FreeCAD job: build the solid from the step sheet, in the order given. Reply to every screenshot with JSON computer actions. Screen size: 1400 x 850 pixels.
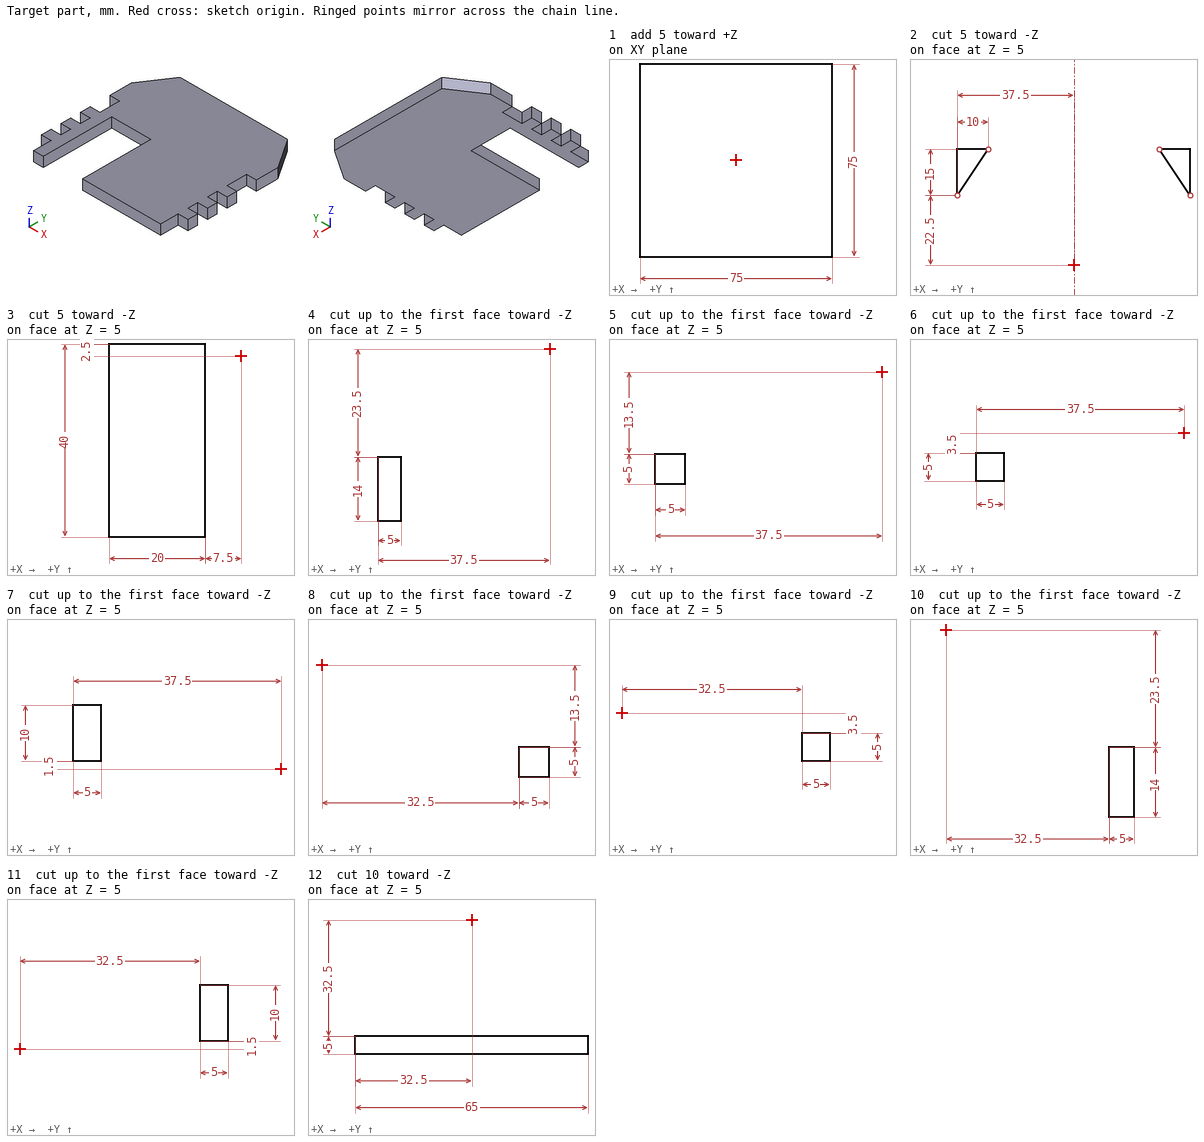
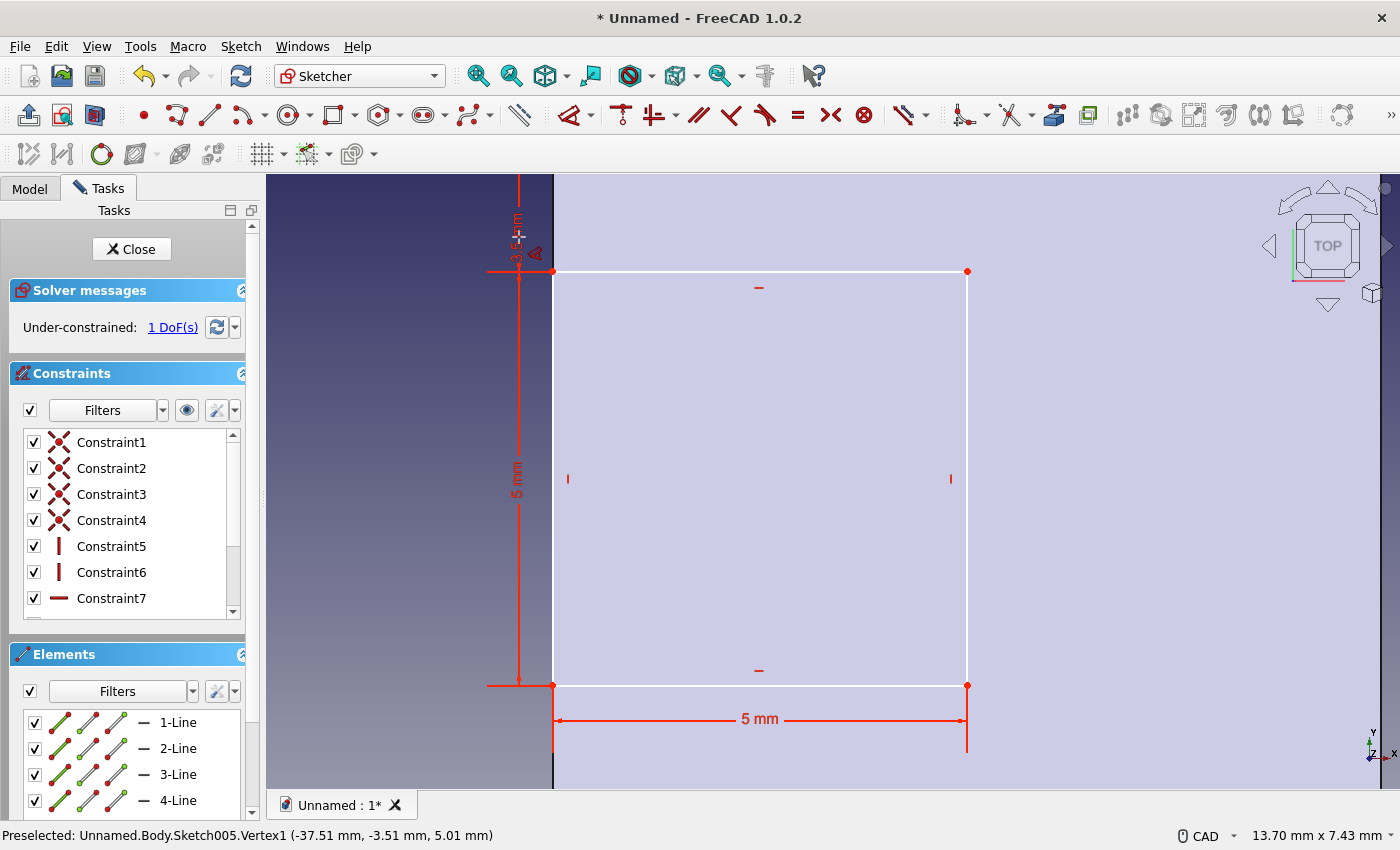
{"action": "left_click", "coordinate": [553, 272]}
{"action": "left_click", "coordinate": [894, 306]}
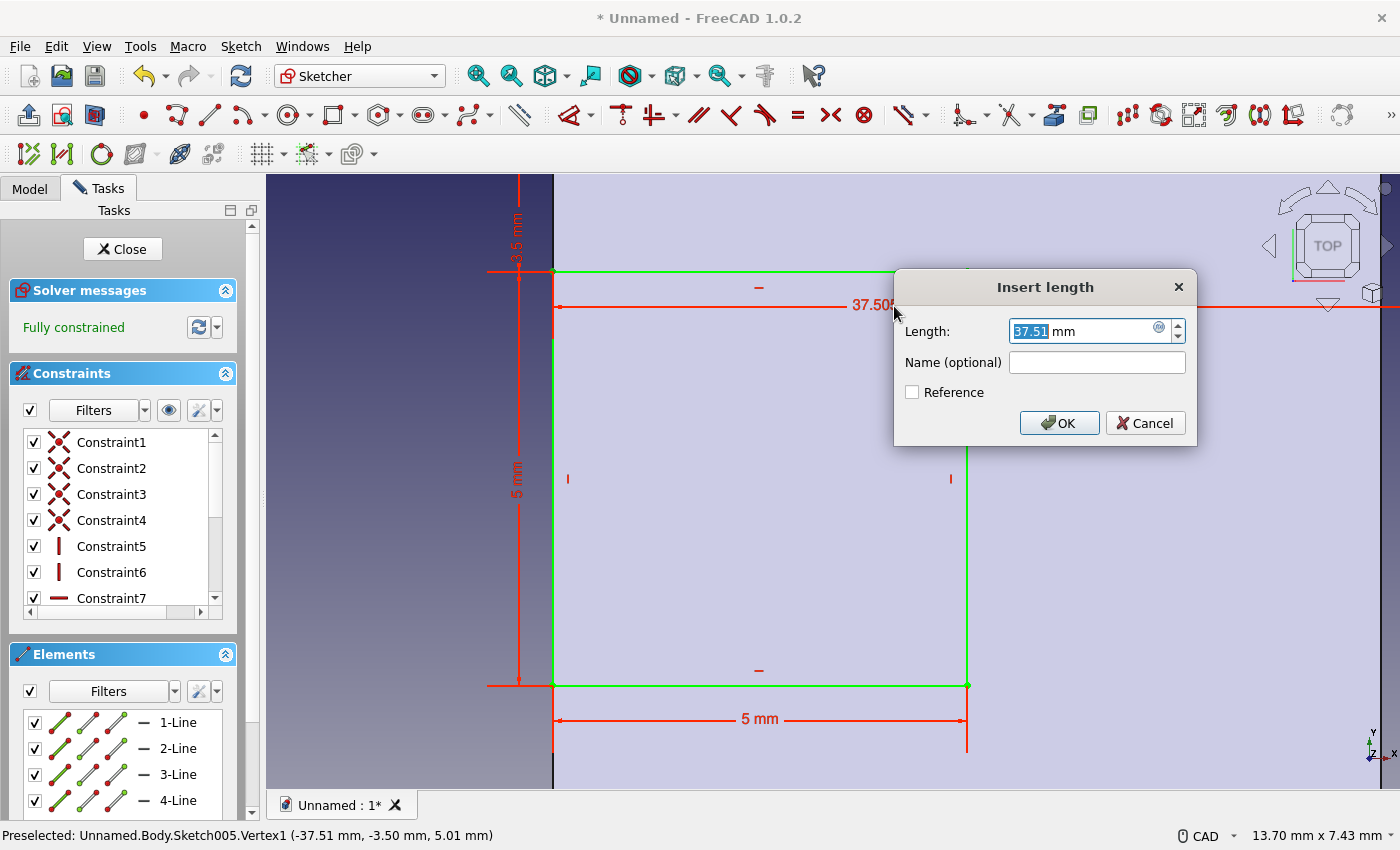
{"action": "type", "text": "37.5"}
{"action": "key", "text": "Return"}
{"action": "key", "text": "Escape"}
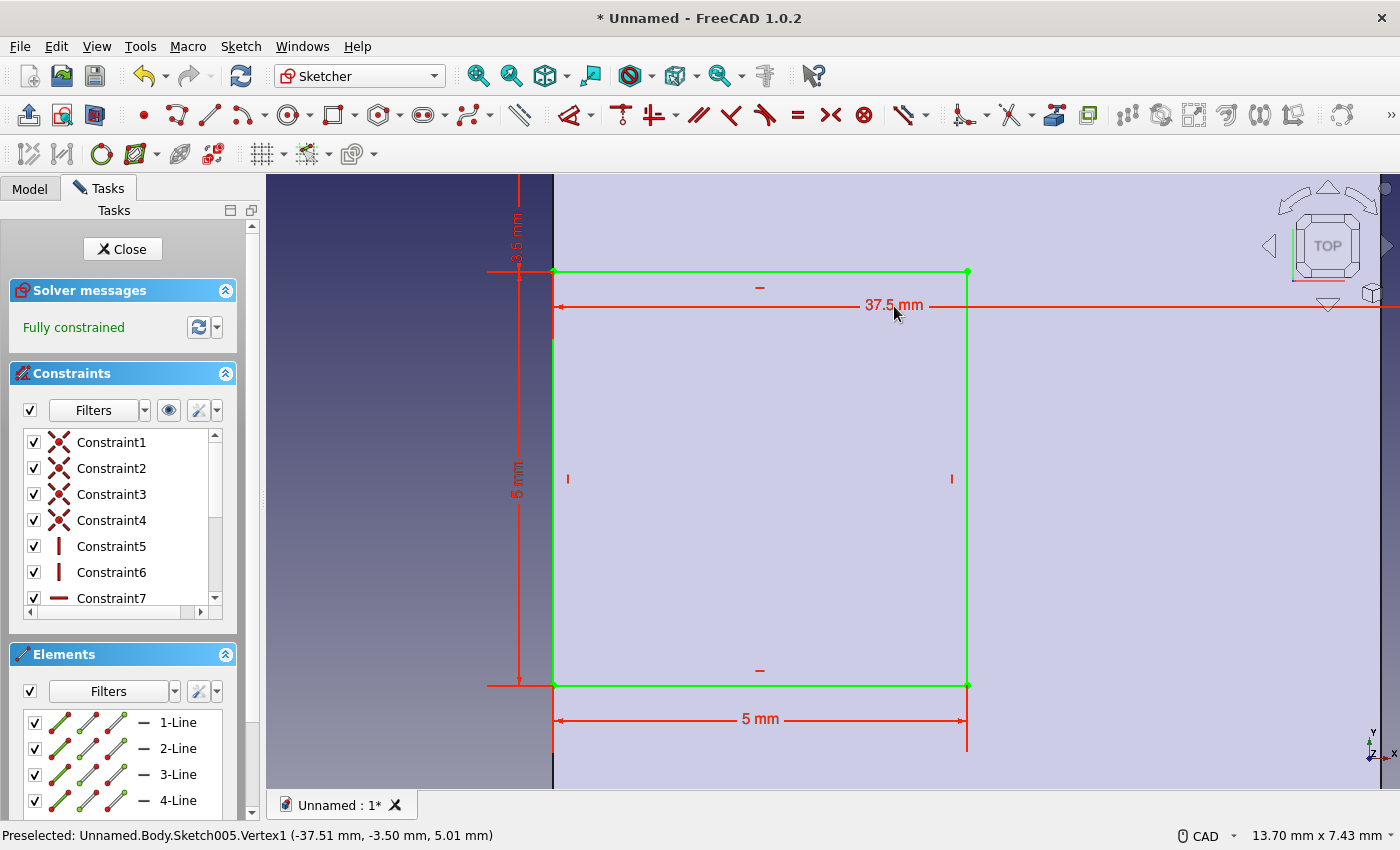
{"action": "left_click", "coordinate": [123, 249]}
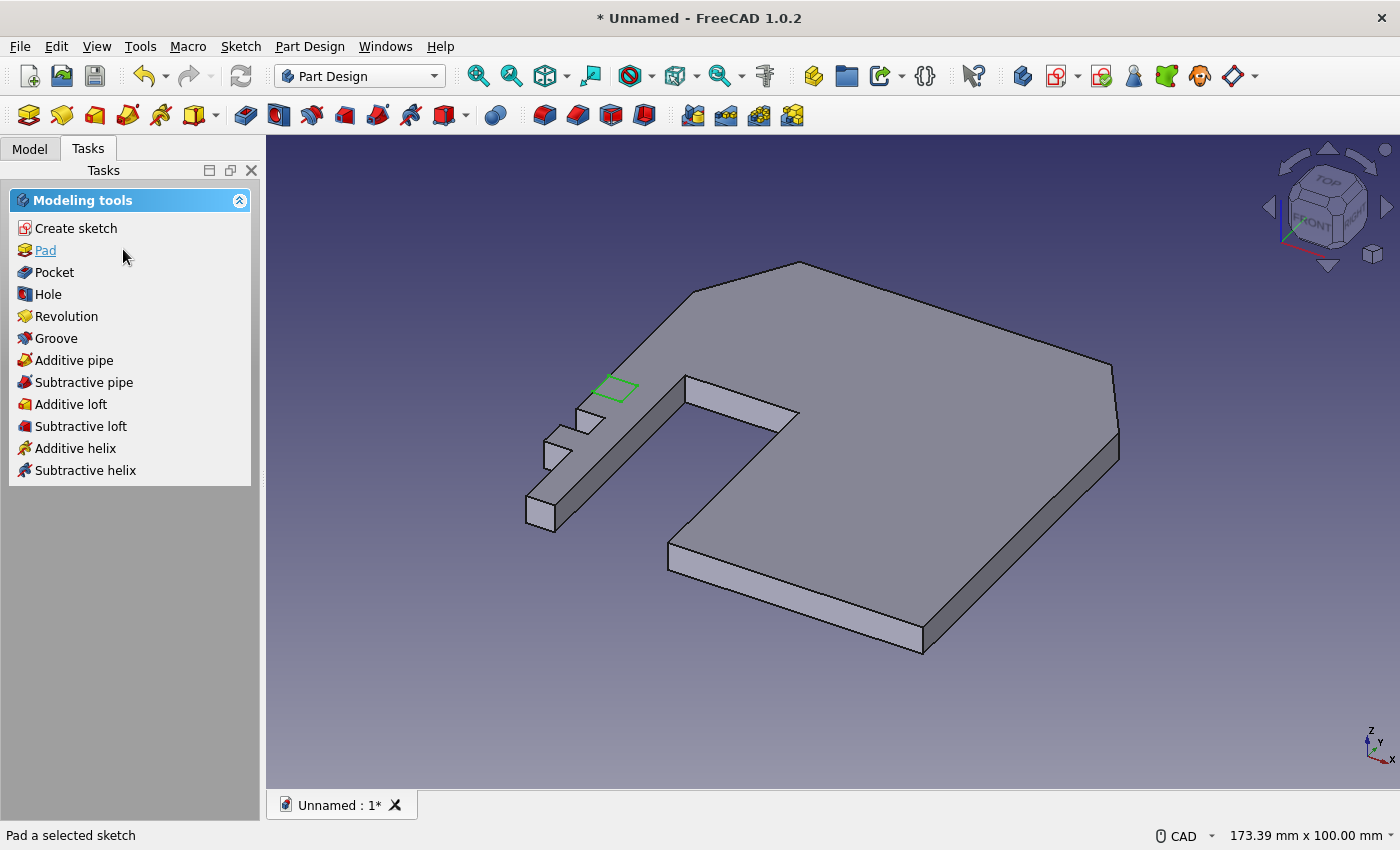
{"action": "left_click", "coordinate": [246, 116]}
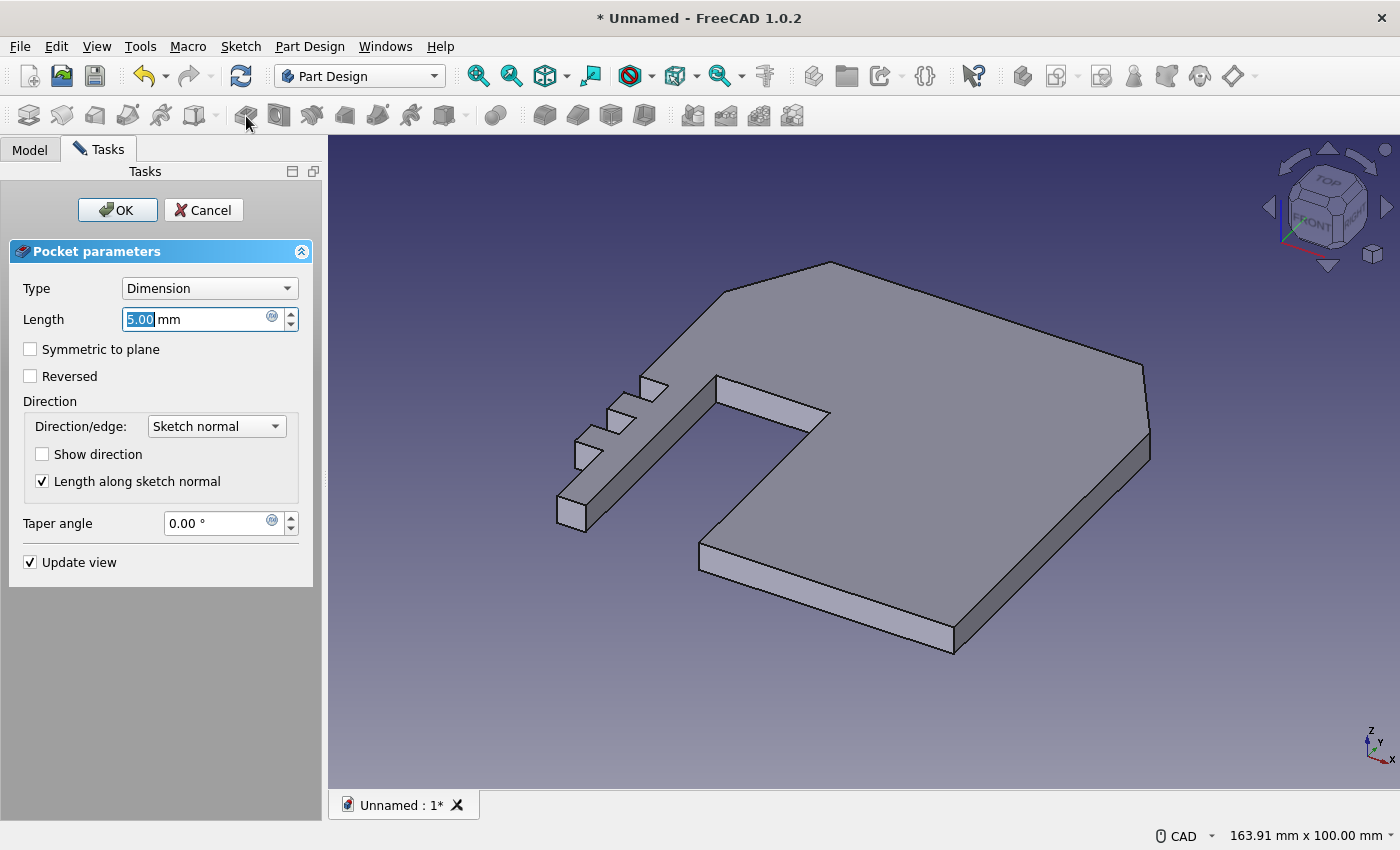
{"action": "left_click", "coordinate": [210, 288]}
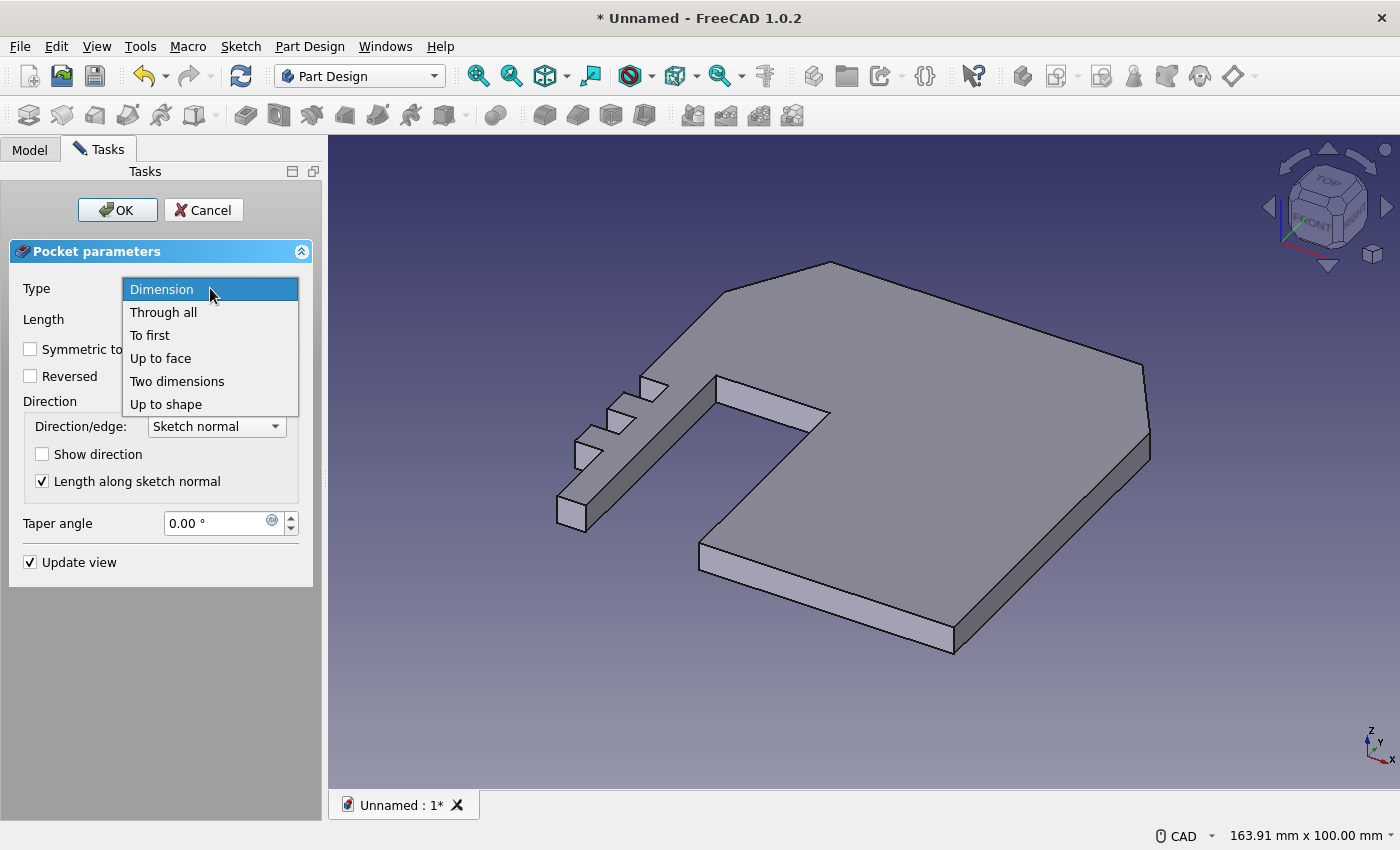
{"action": "left_click", "coordinate": [208, 336]}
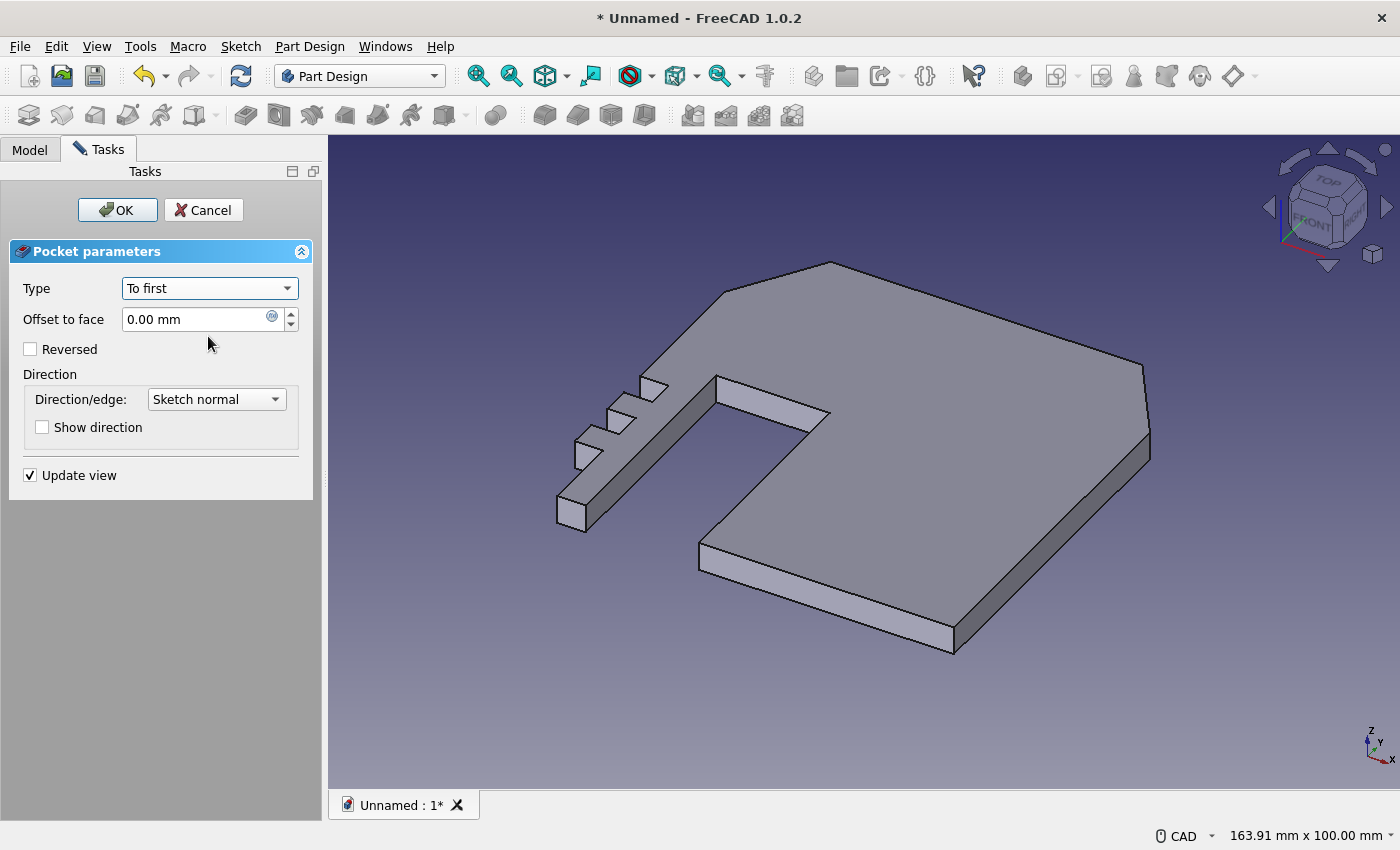
{"action": "left_click", "coordinate": [118, 210]}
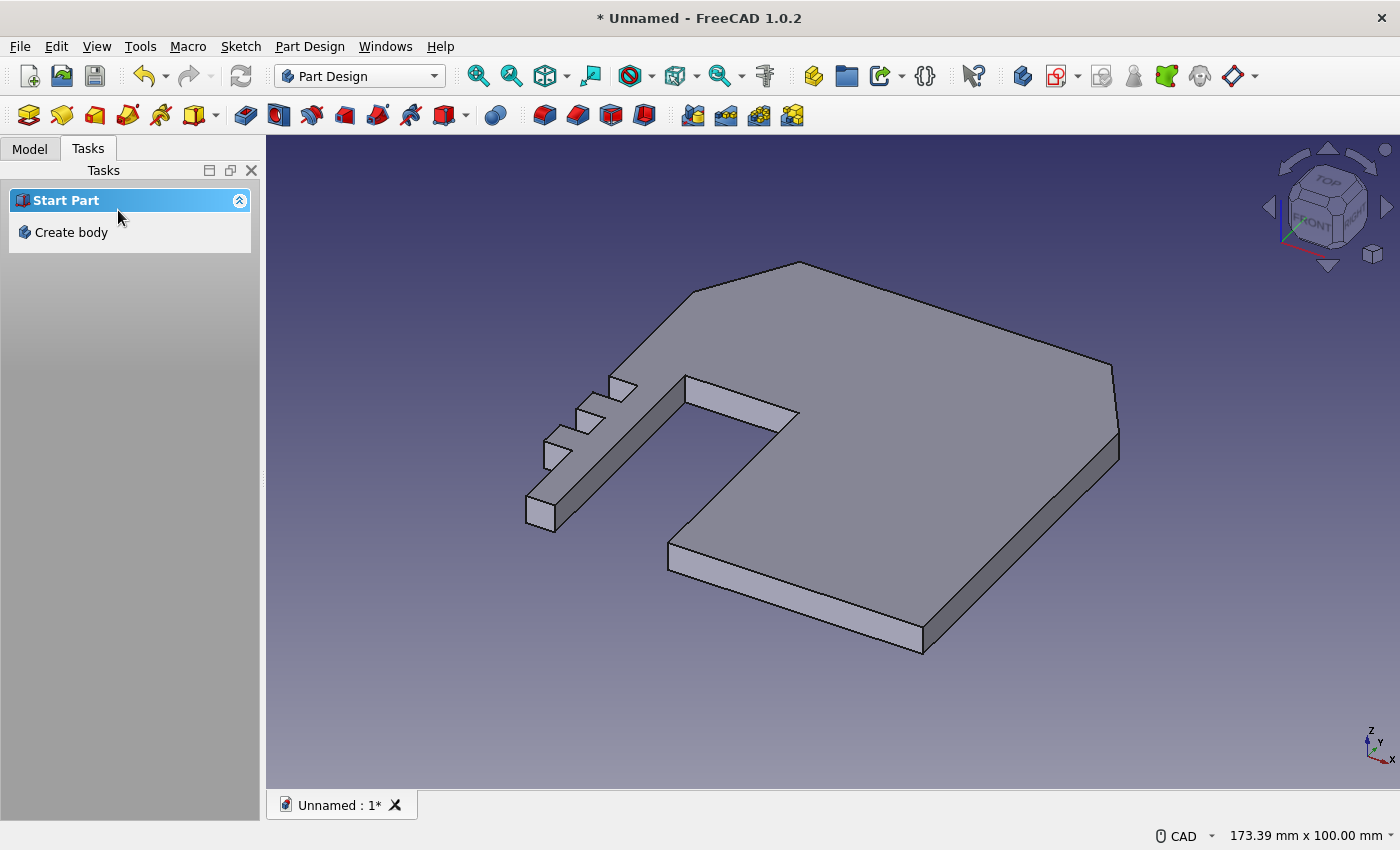
{"action": "left_click", "coordinate": [929, 420]}